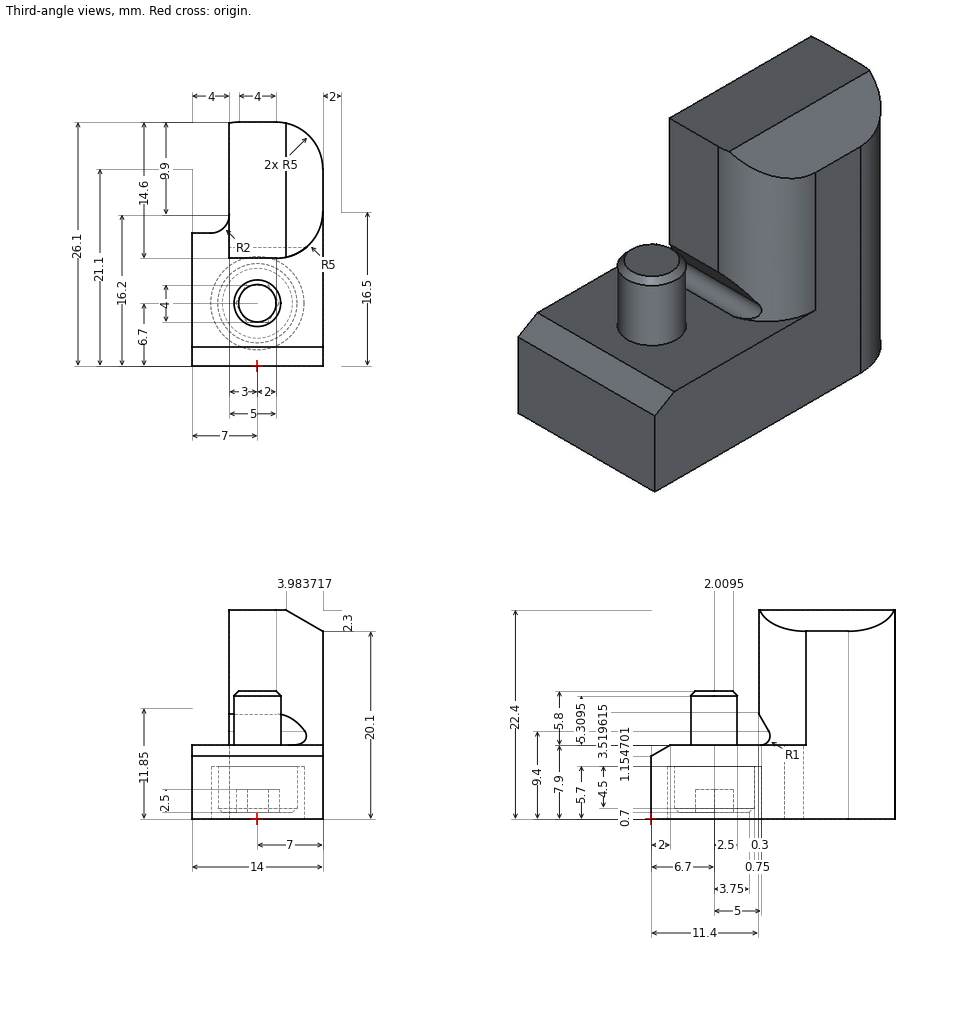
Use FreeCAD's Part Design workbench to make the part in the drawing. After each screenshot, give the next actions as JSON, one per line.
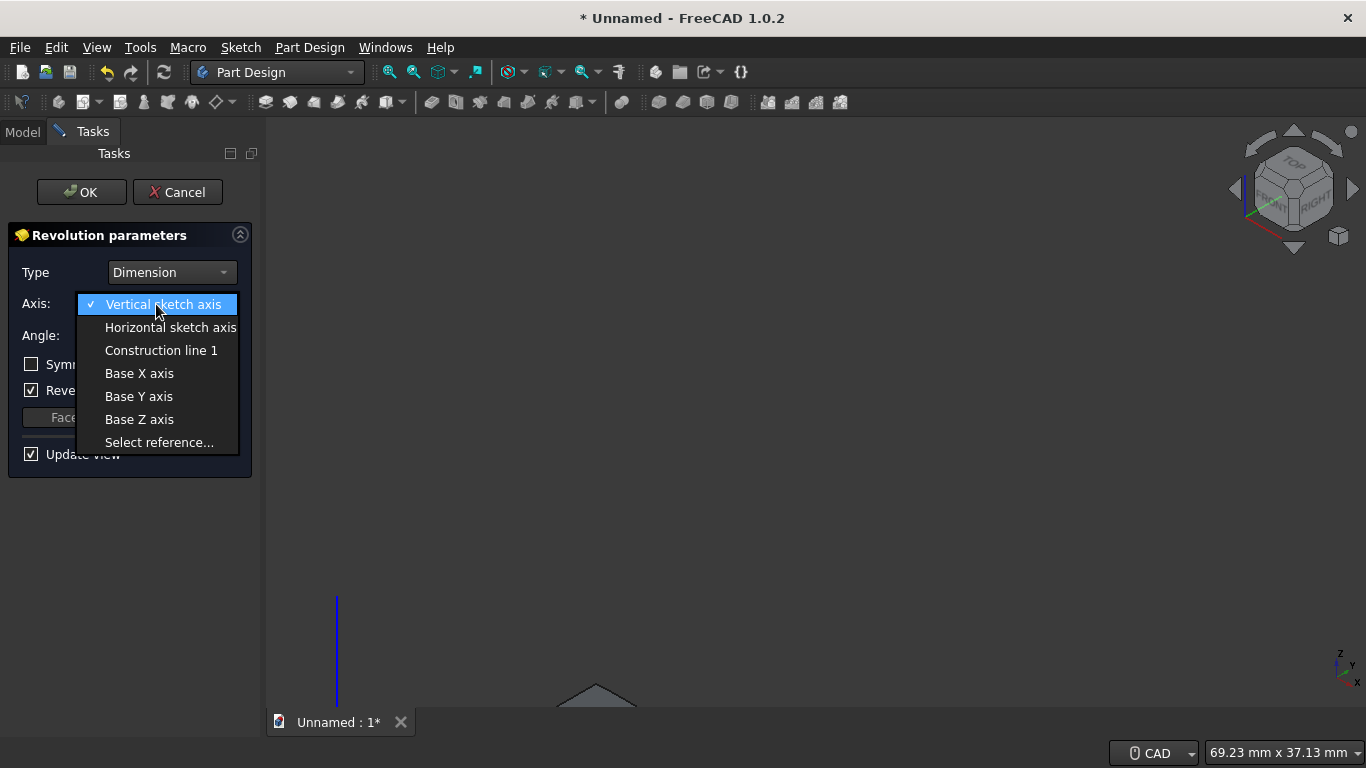
{"action": "left_click", "coordinate": [156, 350]}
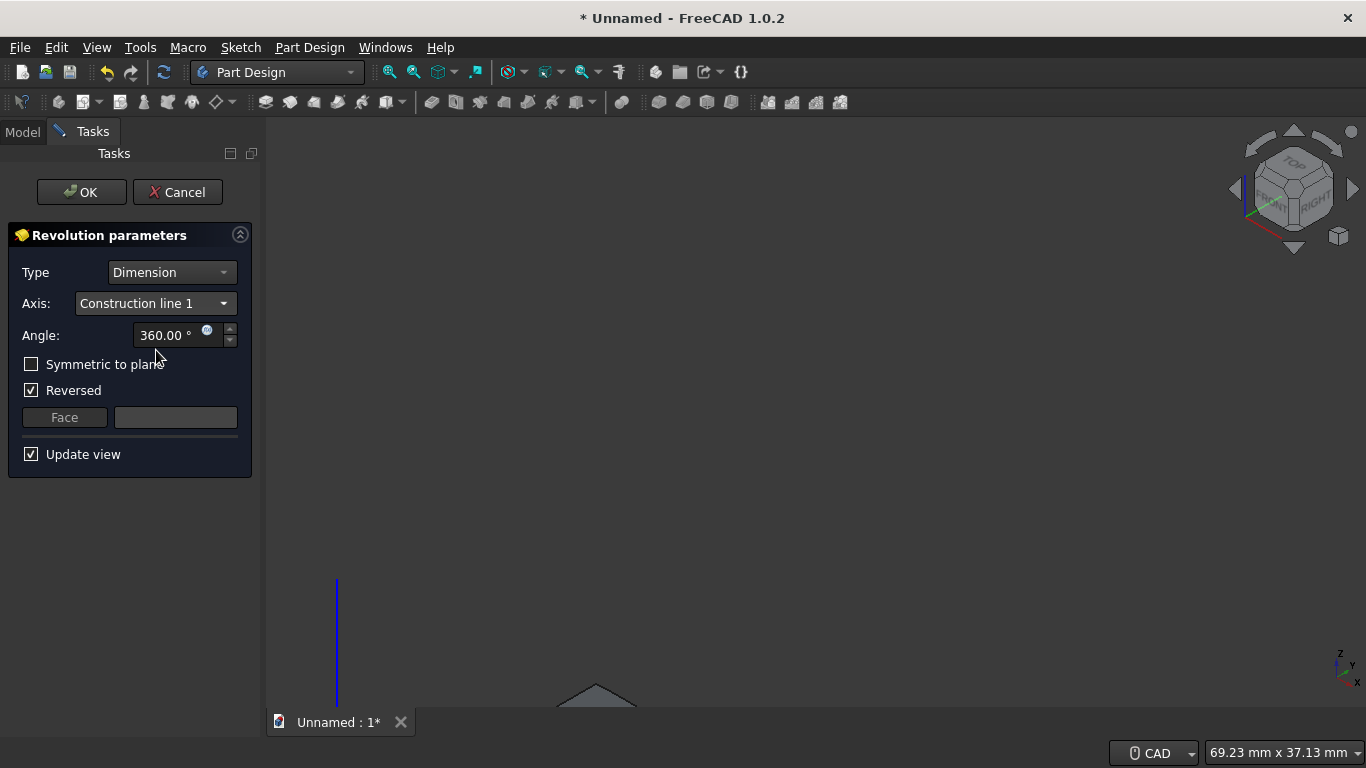
{"action": "left_click", "coordinate": [82, 192]}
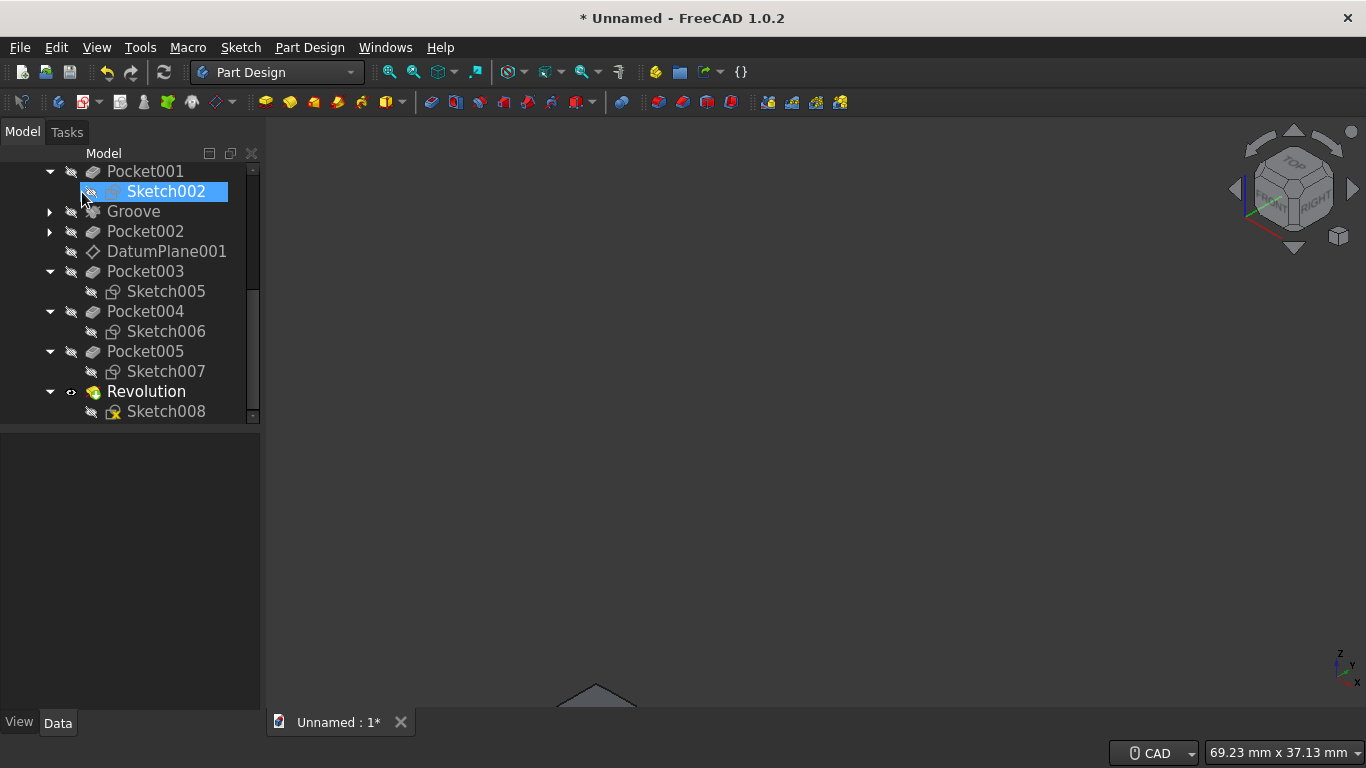
{"action": "left_click", "coordinate": [390, 72]}